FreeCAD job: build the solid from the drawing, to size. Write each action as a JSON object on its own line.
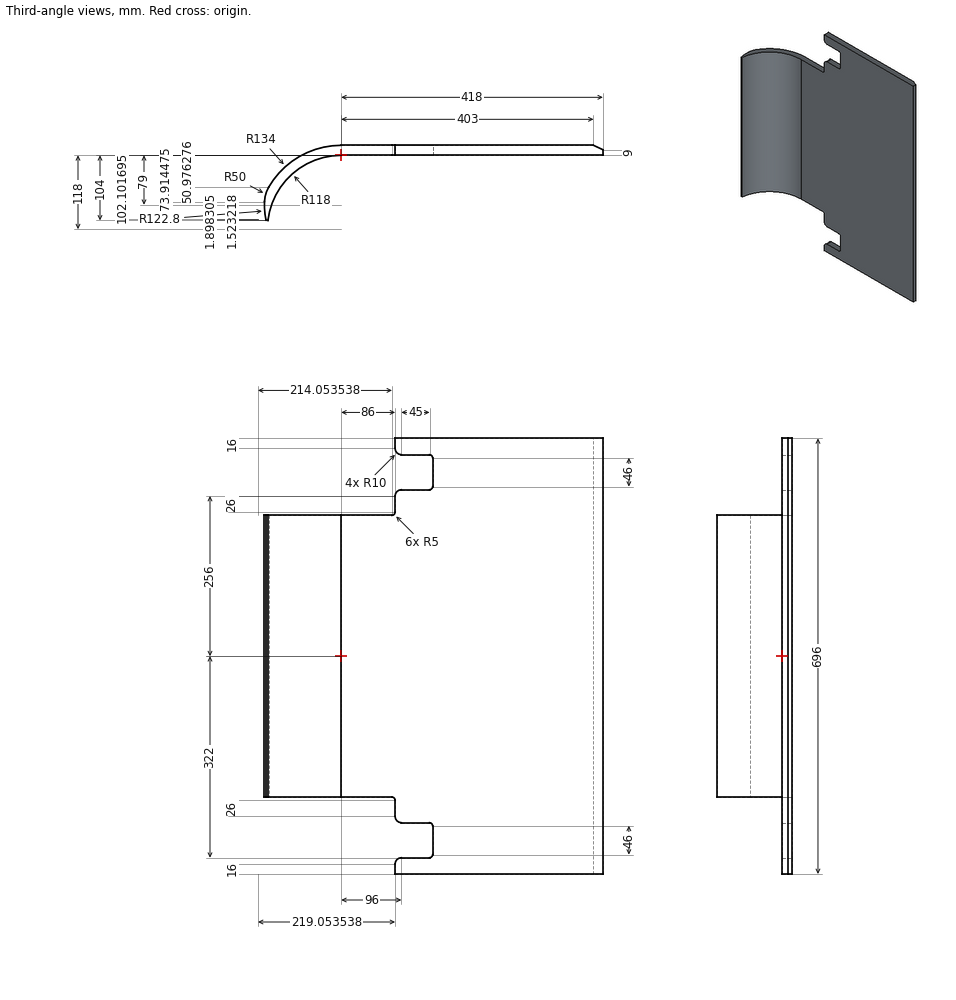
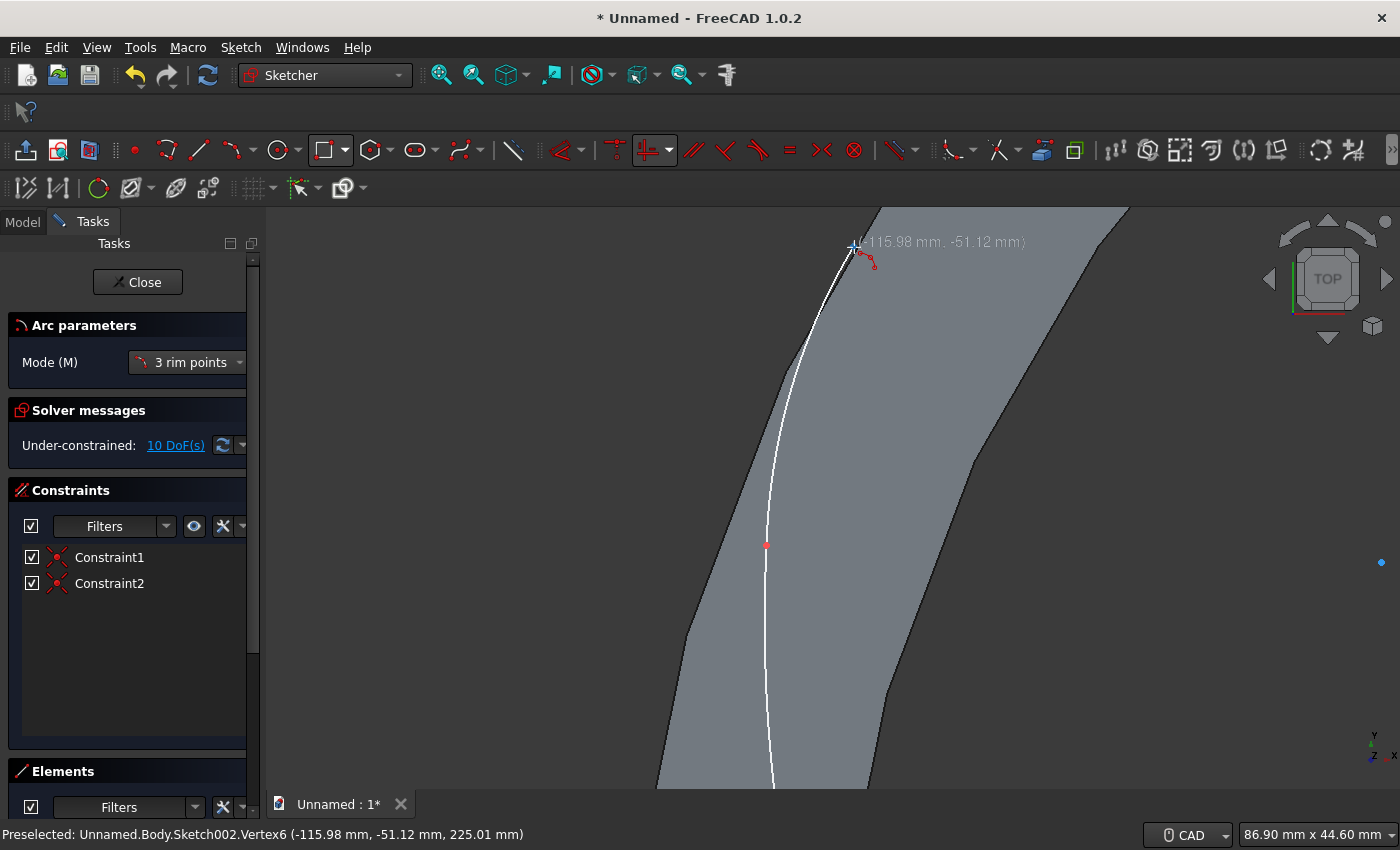
{"action": "scroll", "coordinate": [792, 388], "scroll_direction": "down", "scroll_amount": 3}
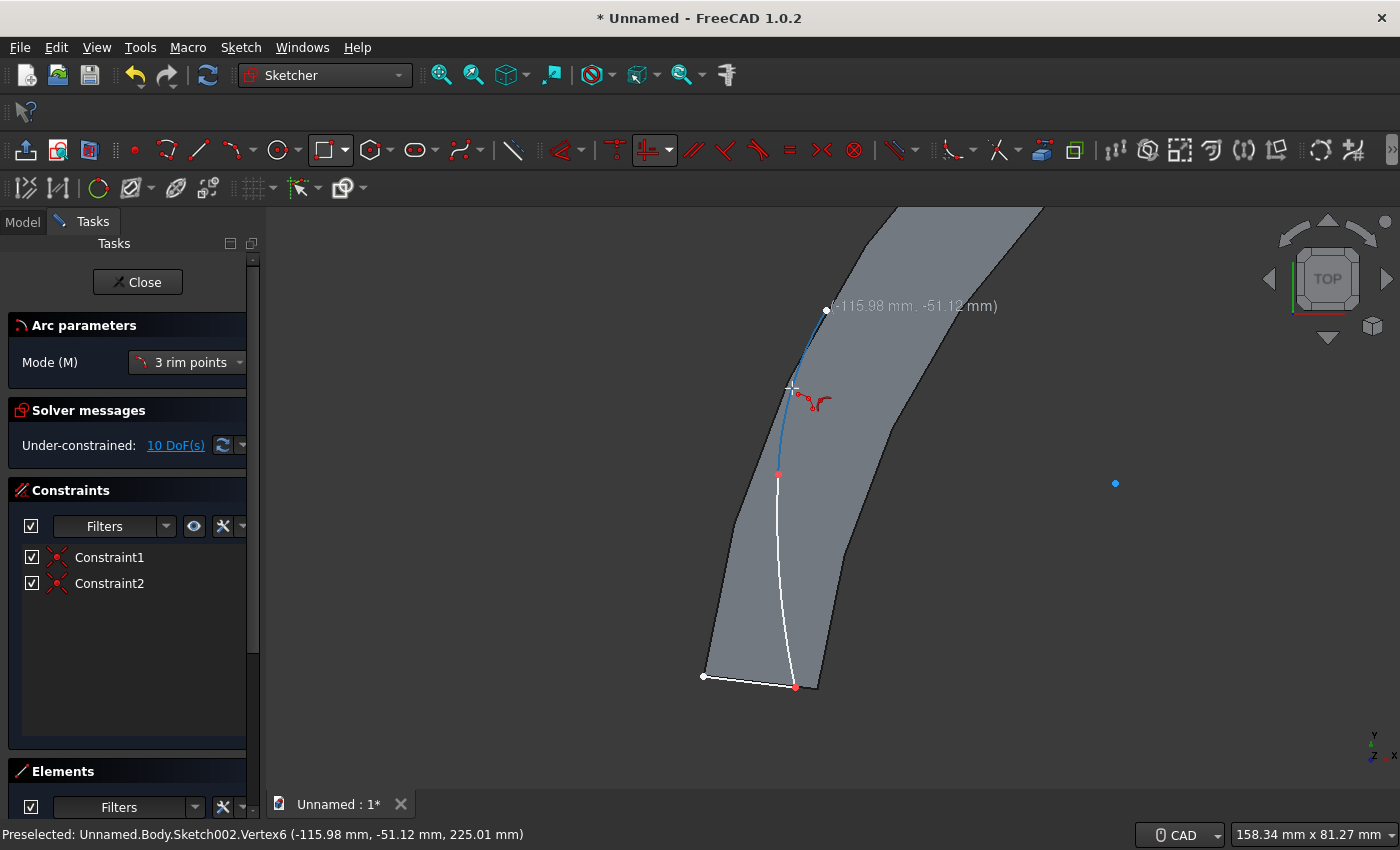
{"action": "left_click", "coordinate": [703, 677]}
{"action": "left_click", "coordinate": [746, 486]}
{"action": "key", "text": "Escape"}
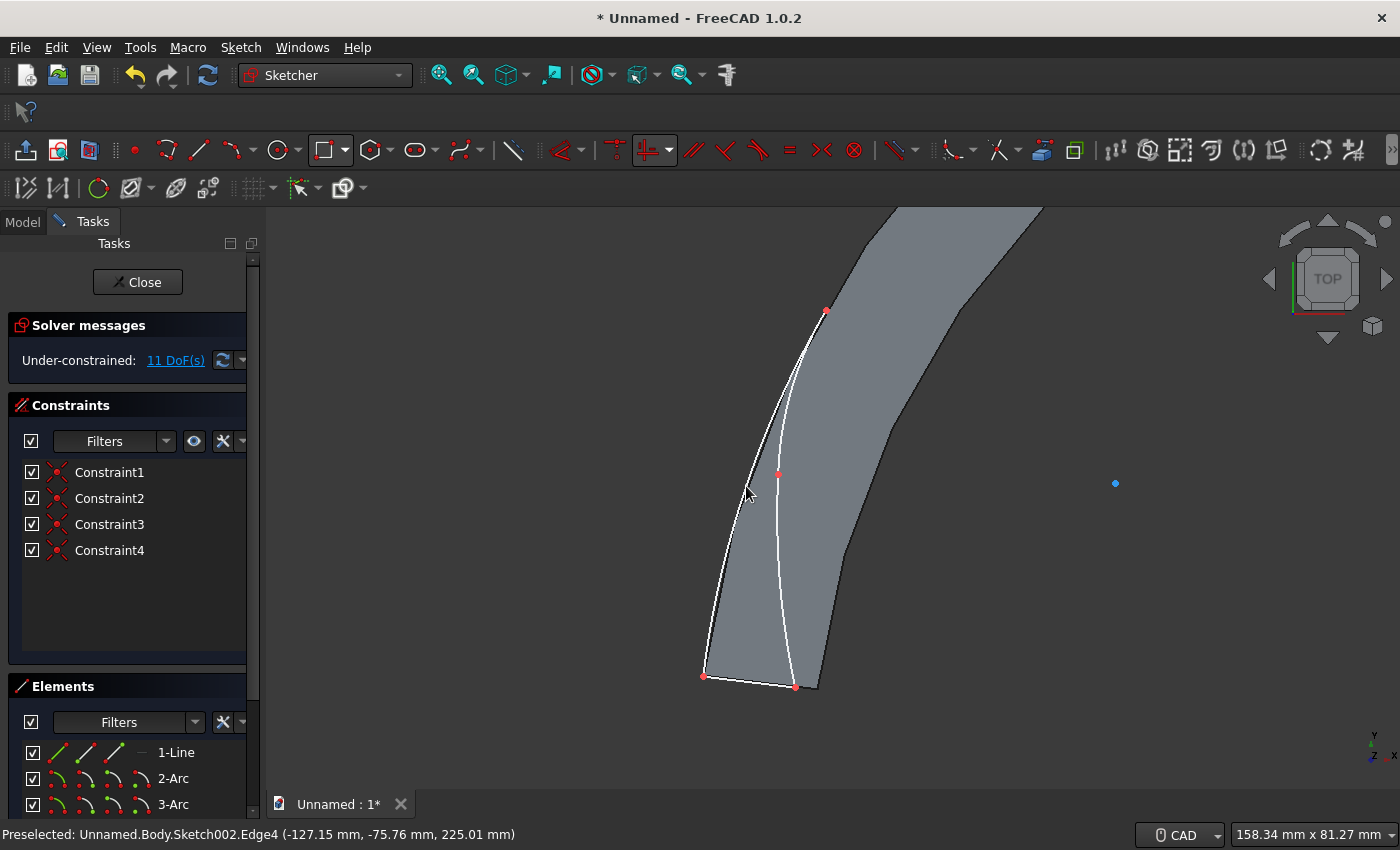
{"action": "scroll", "coordinate": [294, 498], "scroll_direction": "down", "scroll_amount": 2}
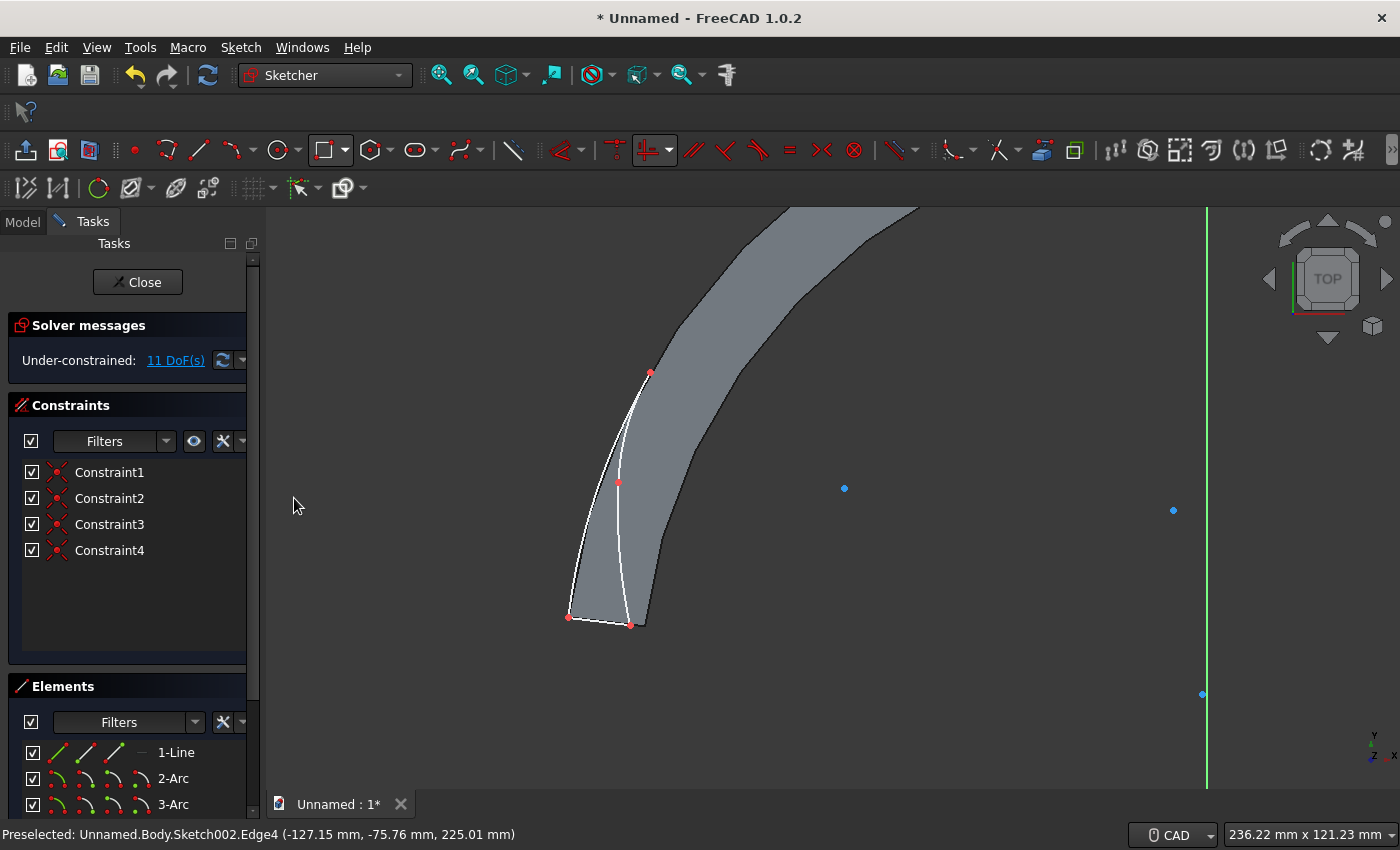
{"action": "left_click", "coordinate": [1173, 510]}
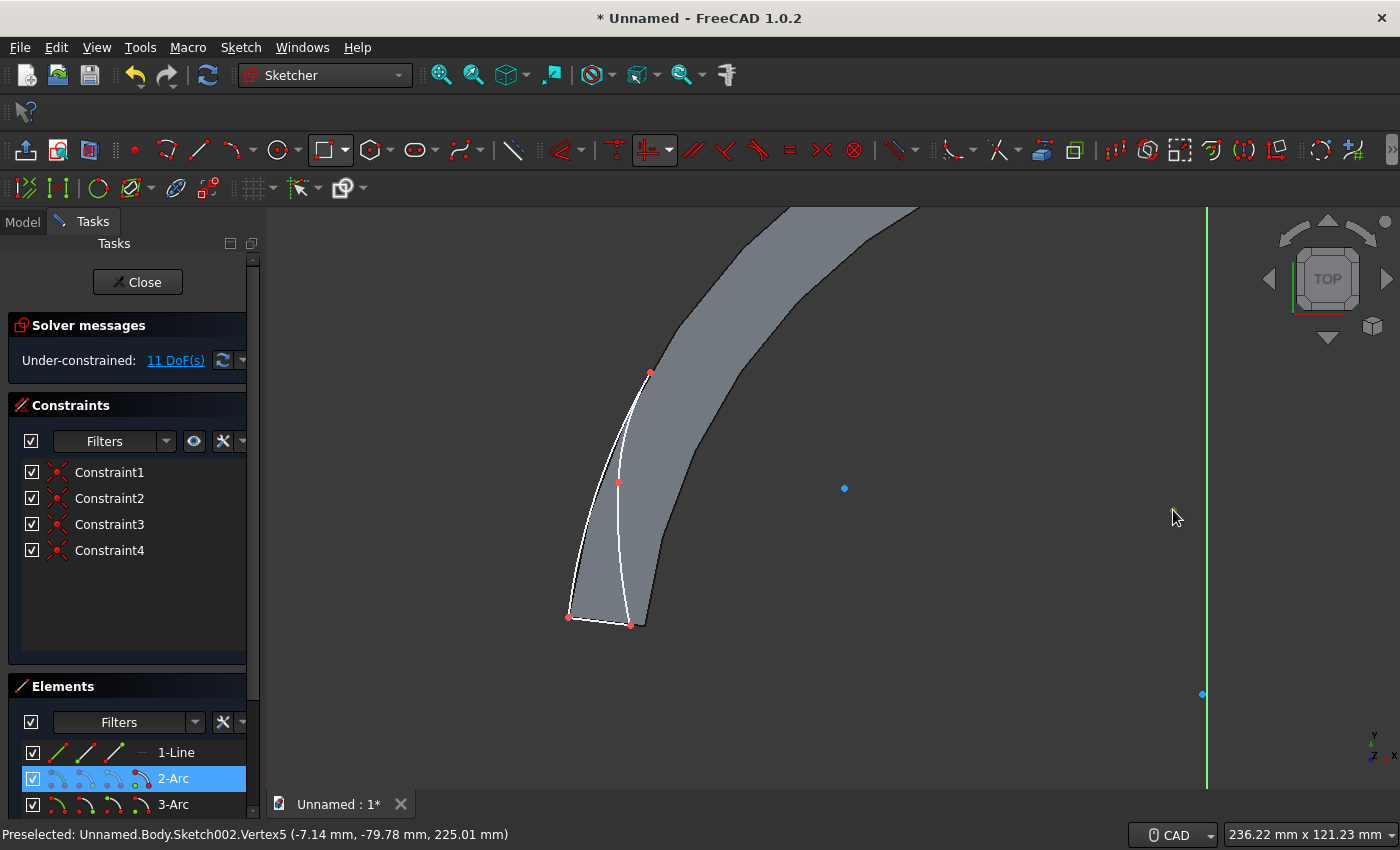
{"action": "left_click", "coordinate": [1207, 723]}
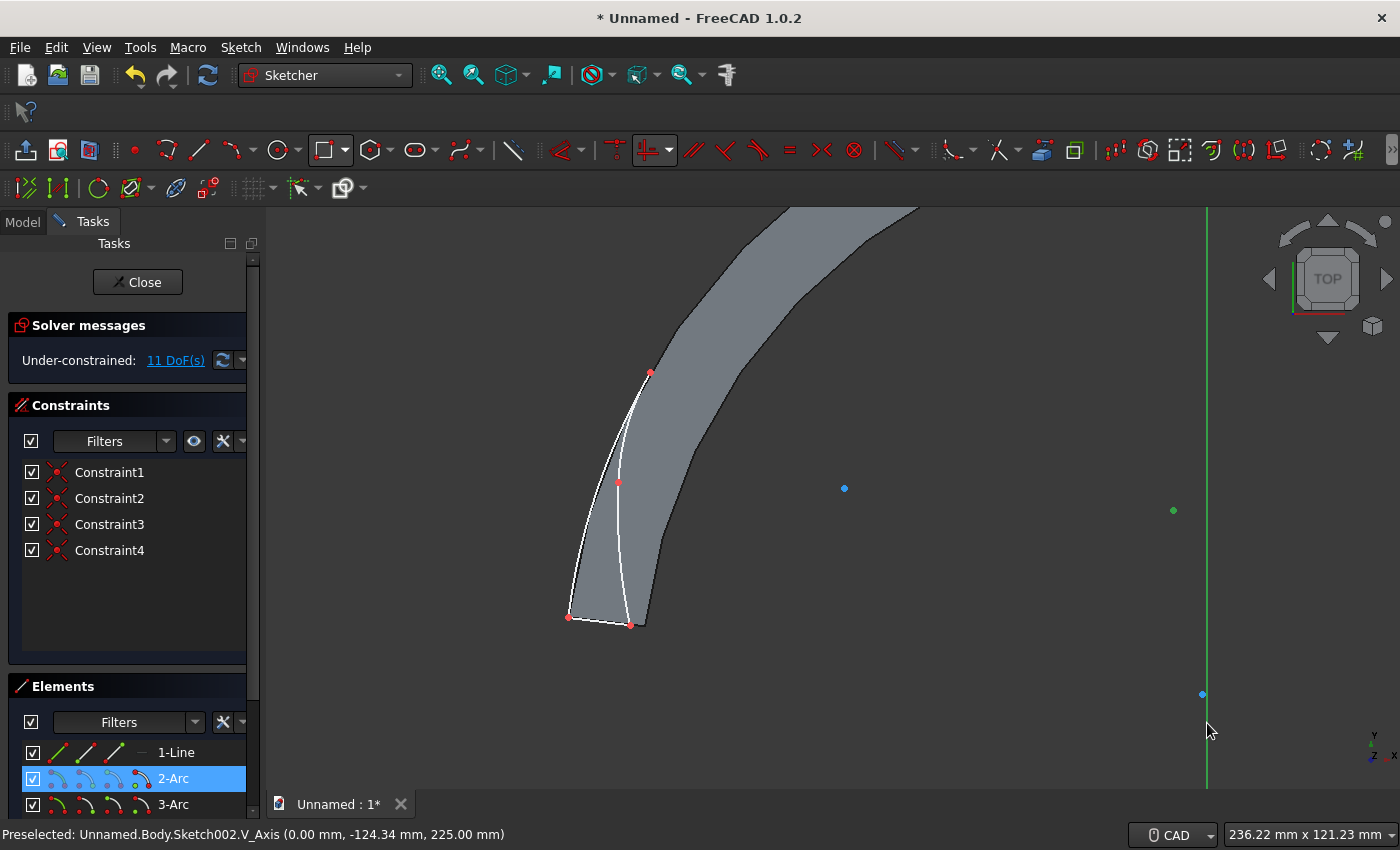
{"action": "left_click", "coordinate": [616, 150]}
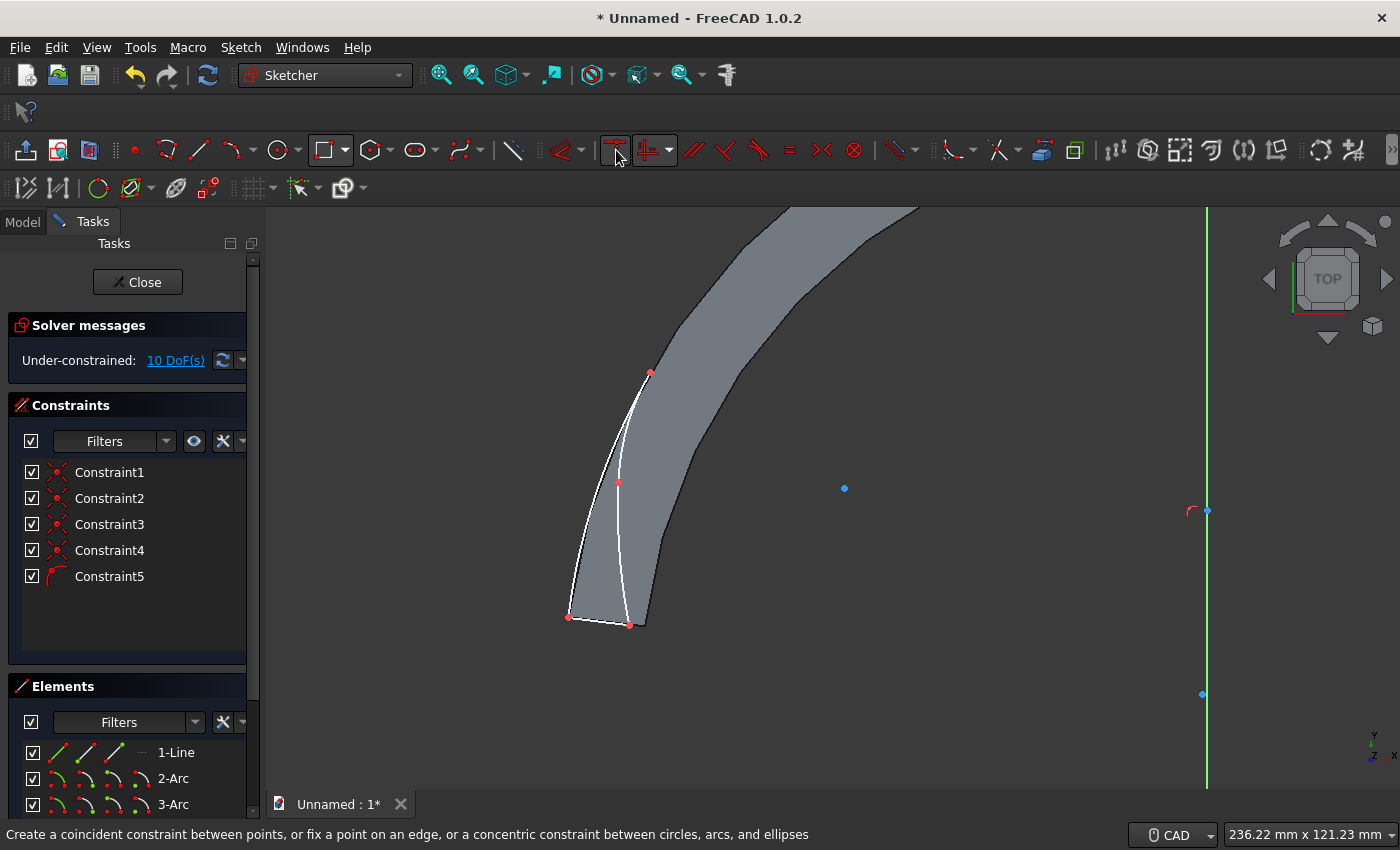
{"action": "left_click", "coordinate": [1203, 694]}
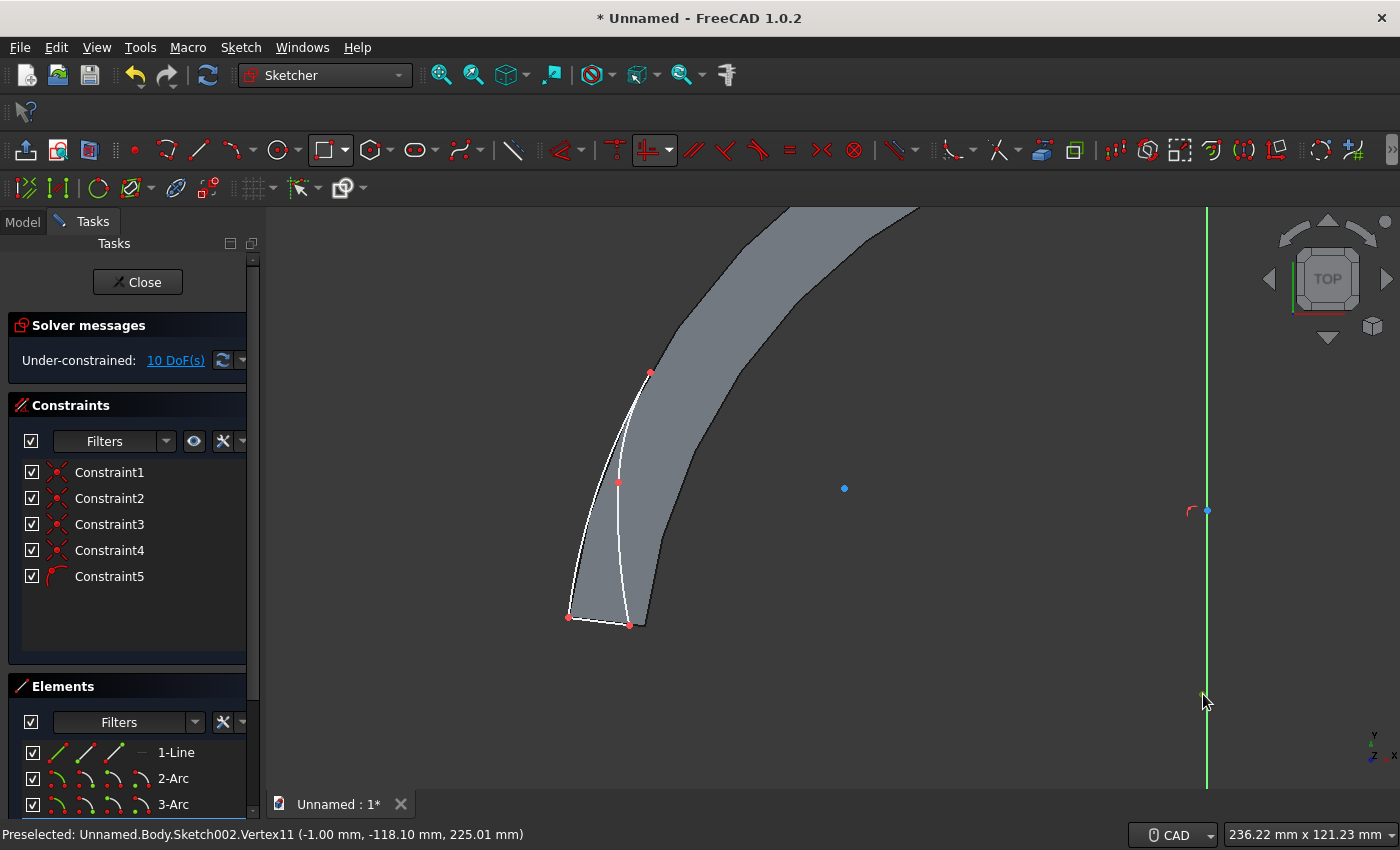
{"action": "left_click", "coordinate": [1207, 723]}